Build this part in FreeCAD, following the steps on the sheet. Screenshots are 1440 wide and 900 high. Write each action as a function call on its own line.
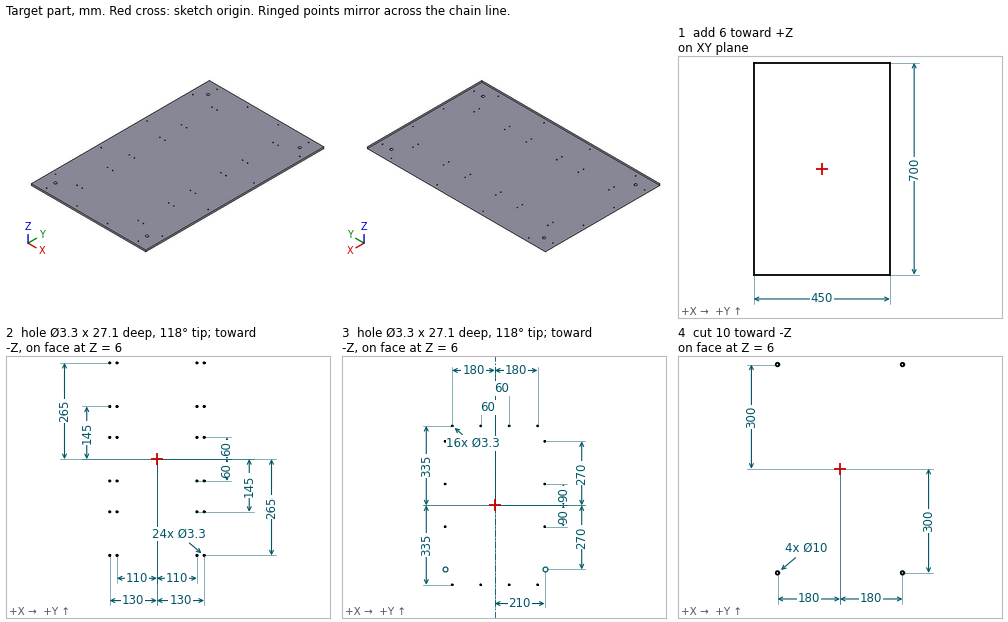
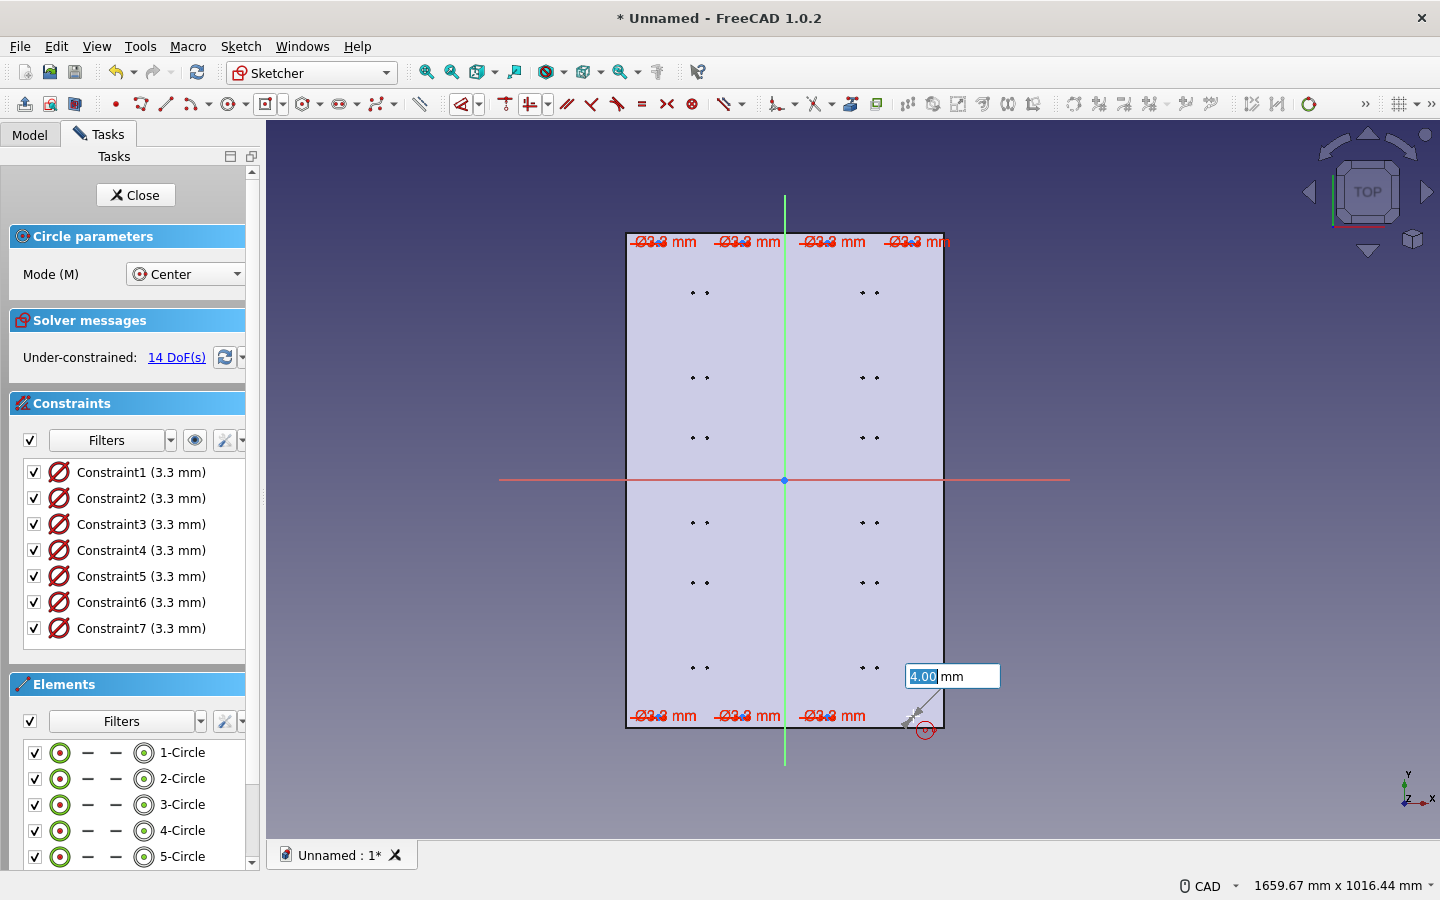
text(3.3)
key(Return)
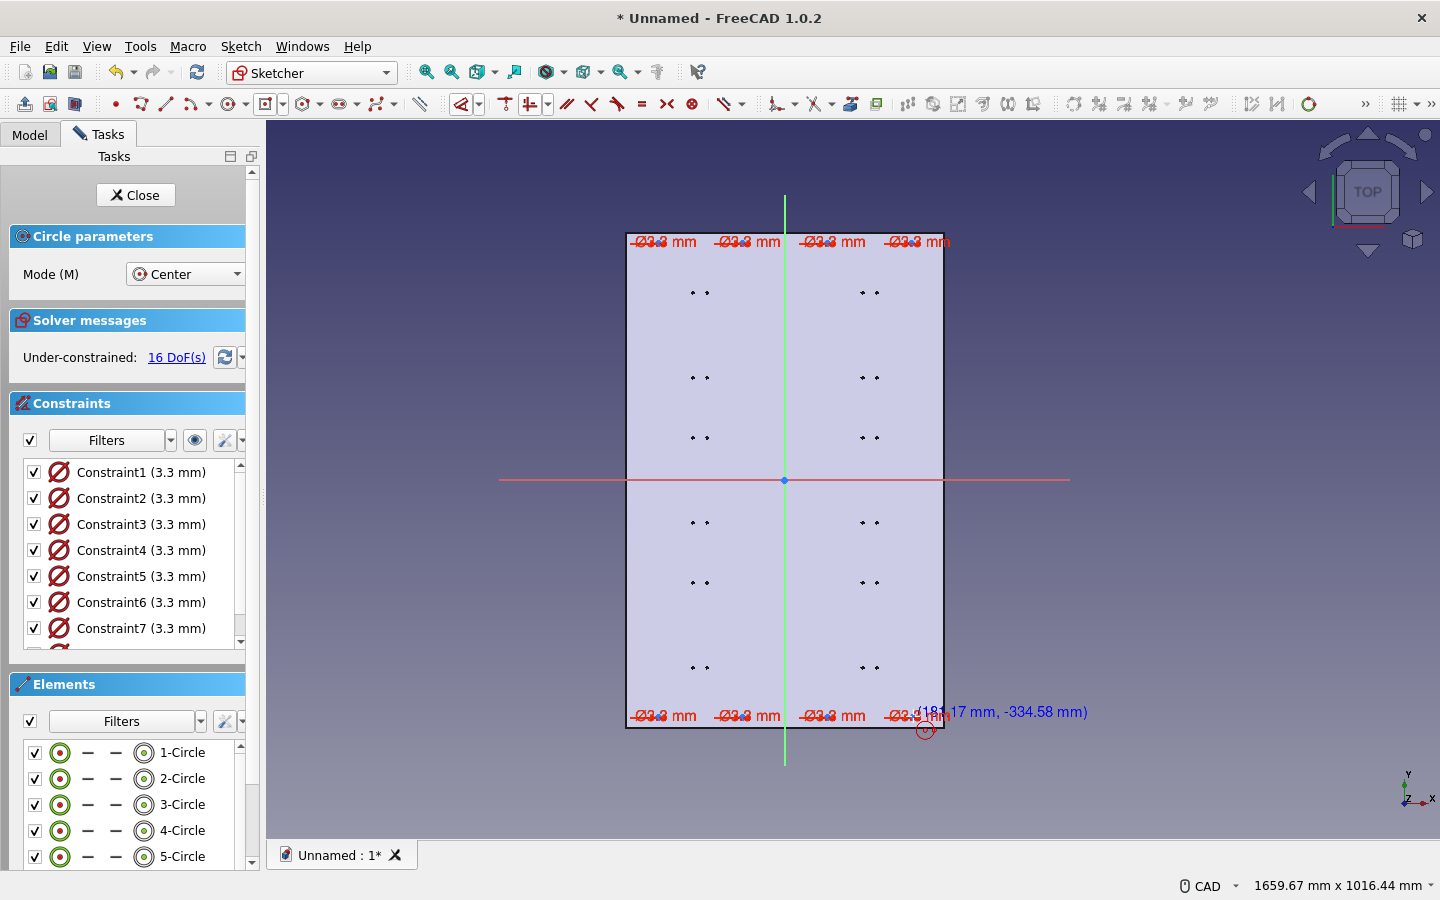
scroll(933, 671, up, 15)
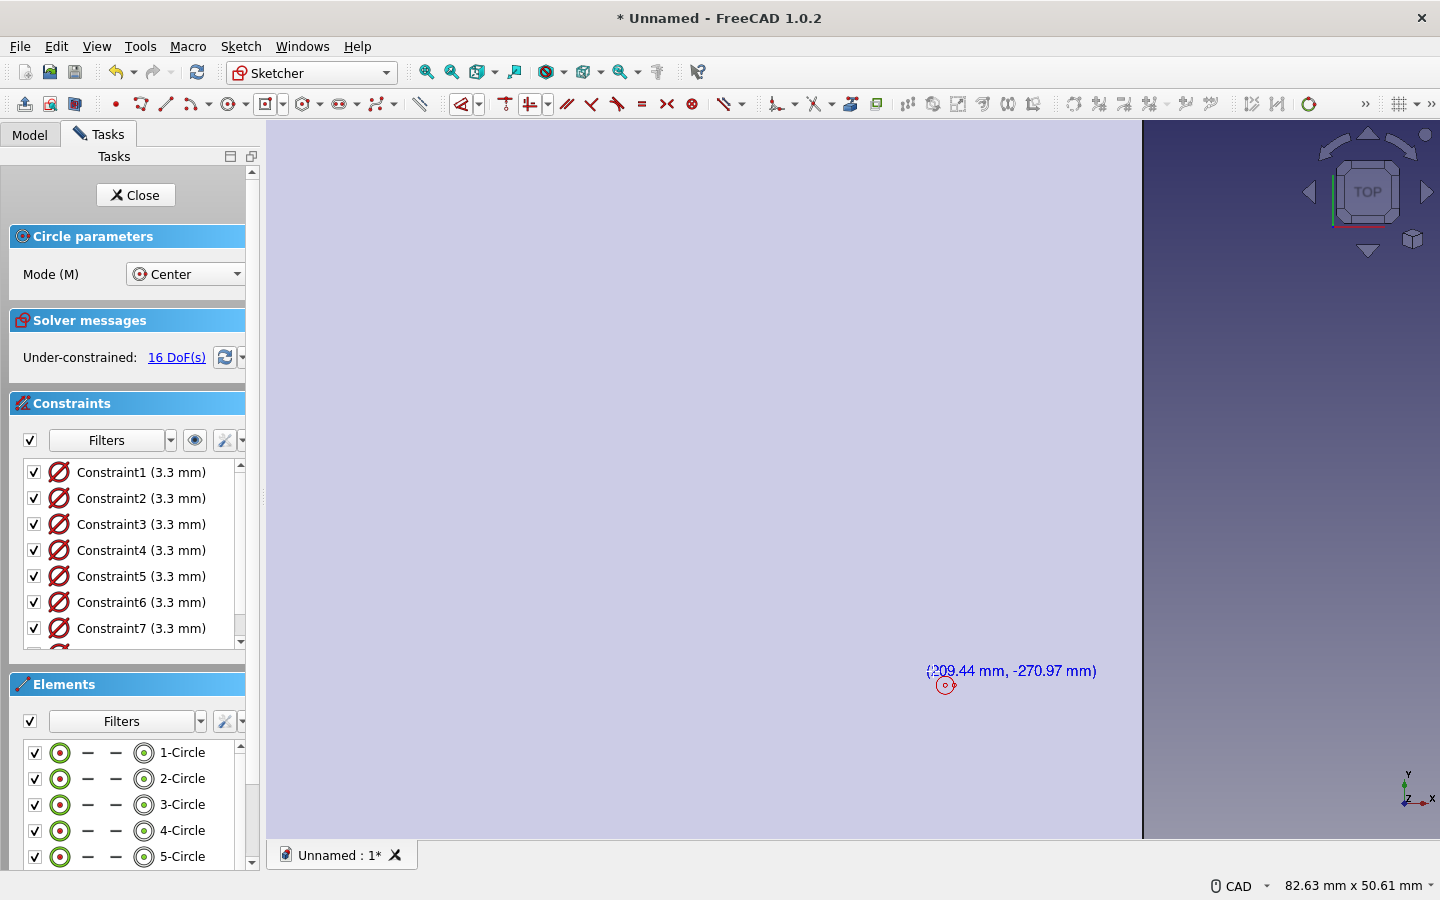
scroll(933, 671, down, 15)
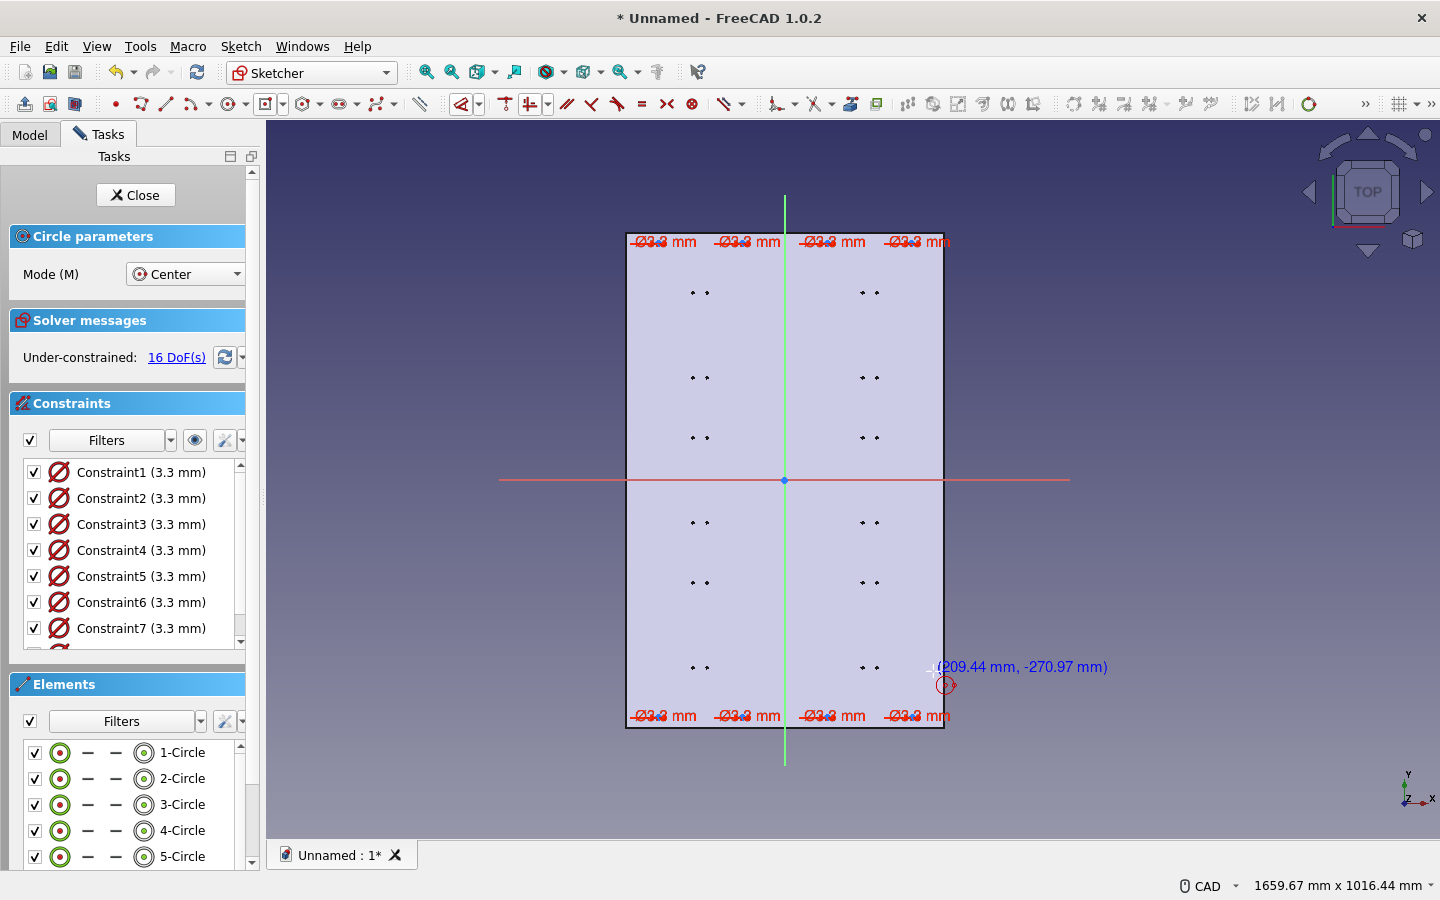
click(933, 671)
move(934, 670)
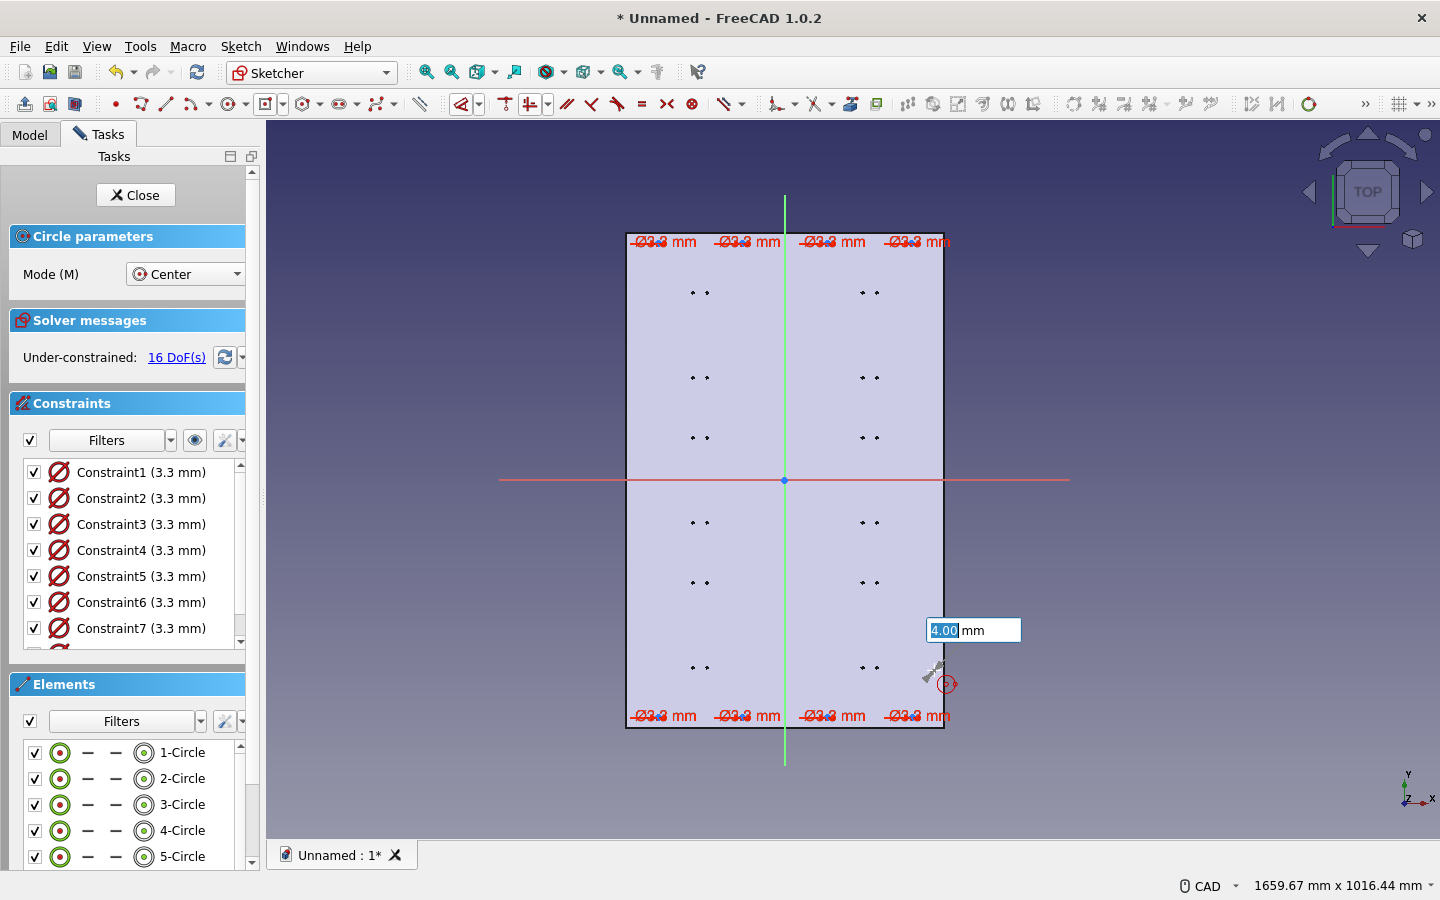
text(3.3)
key(Return)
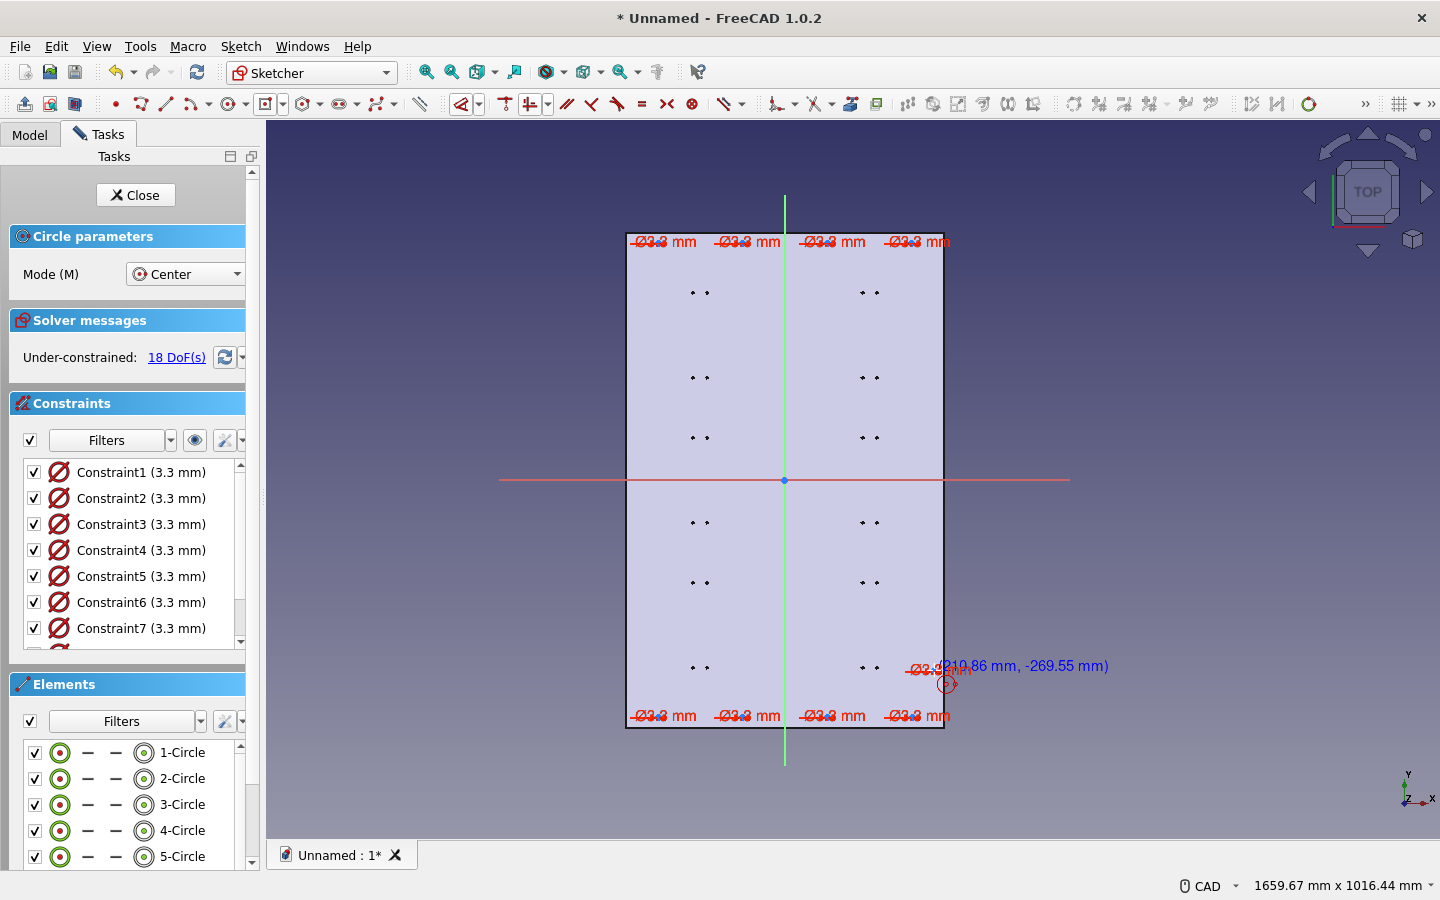
scroll(933, 544, up, 15)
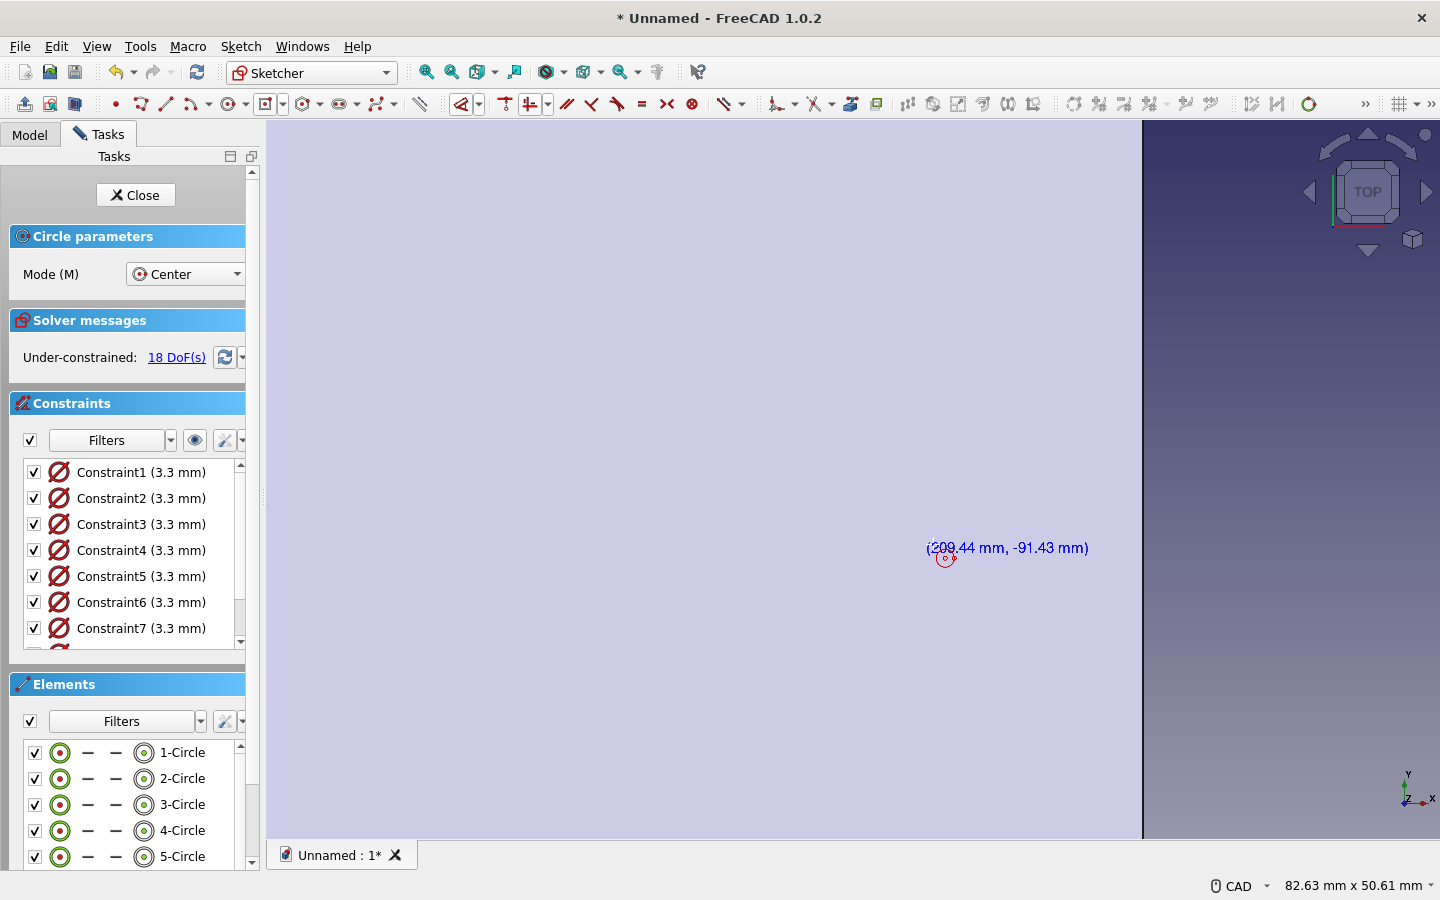
scroll(933, 544, down, 15)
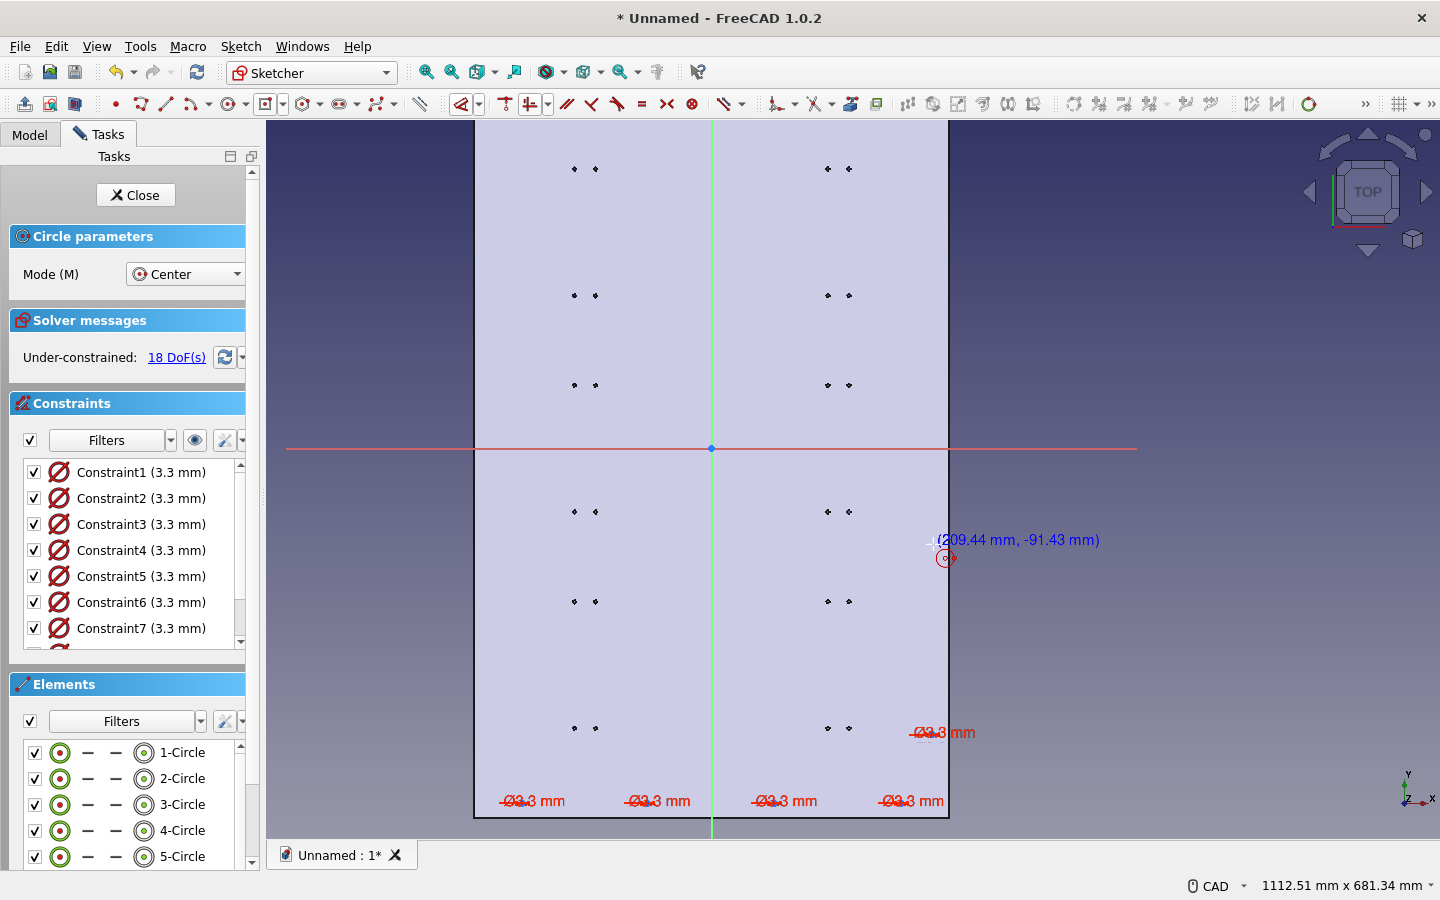
click(933, 544)
move(934, 543)